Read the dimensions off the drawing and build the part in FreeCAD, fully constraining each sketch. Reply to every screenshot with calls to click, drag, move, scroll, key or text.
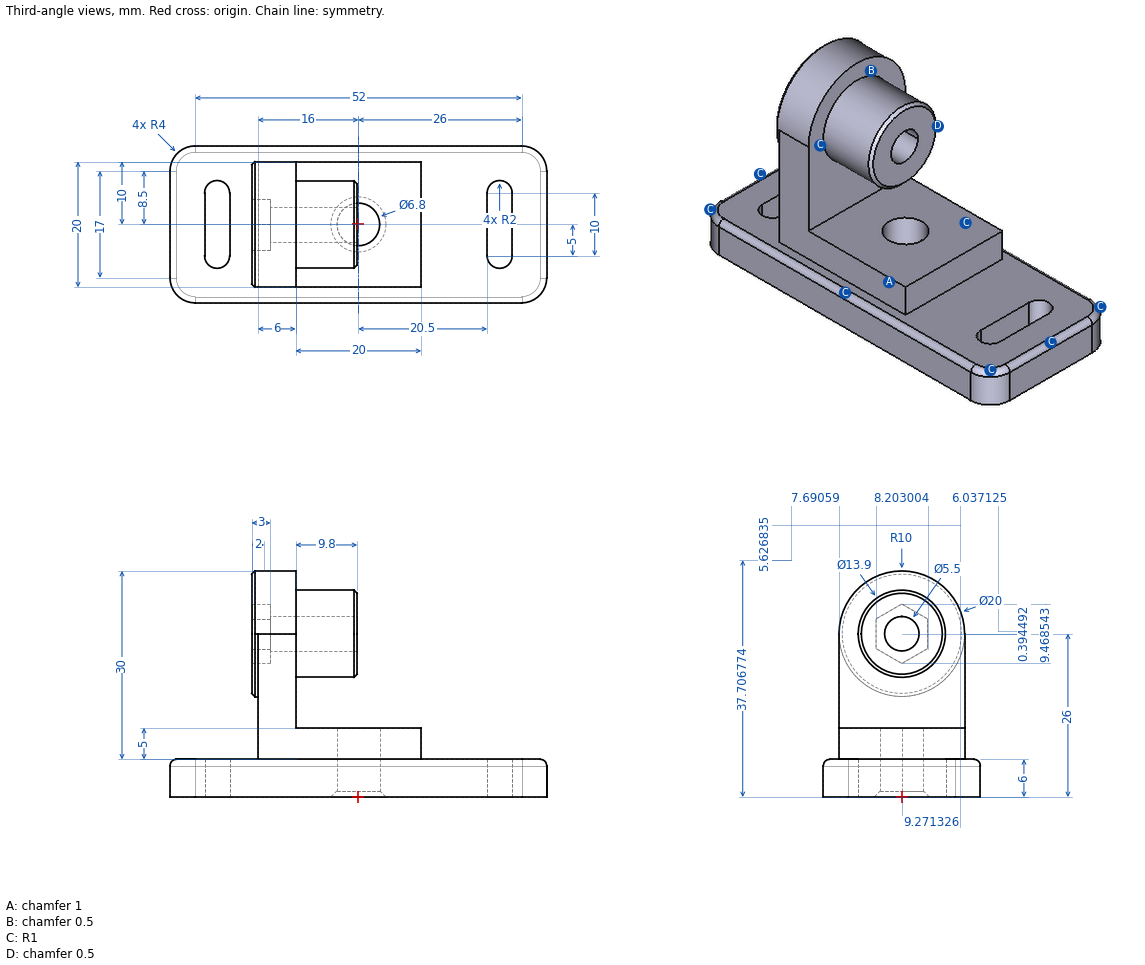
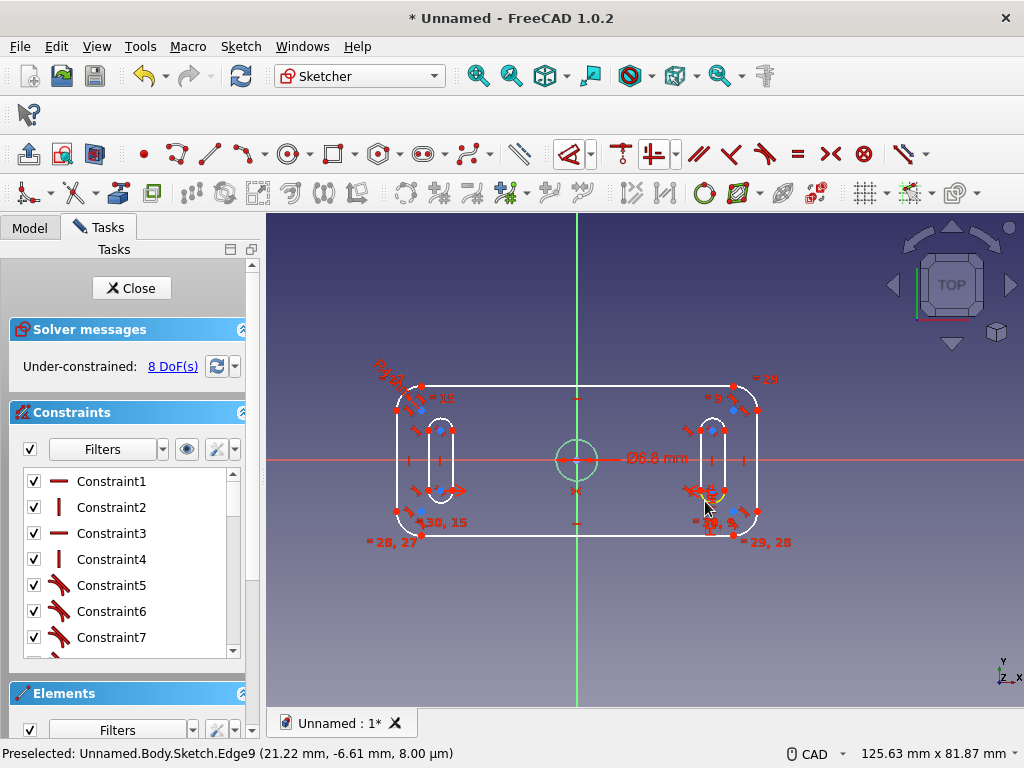
click(639, 386)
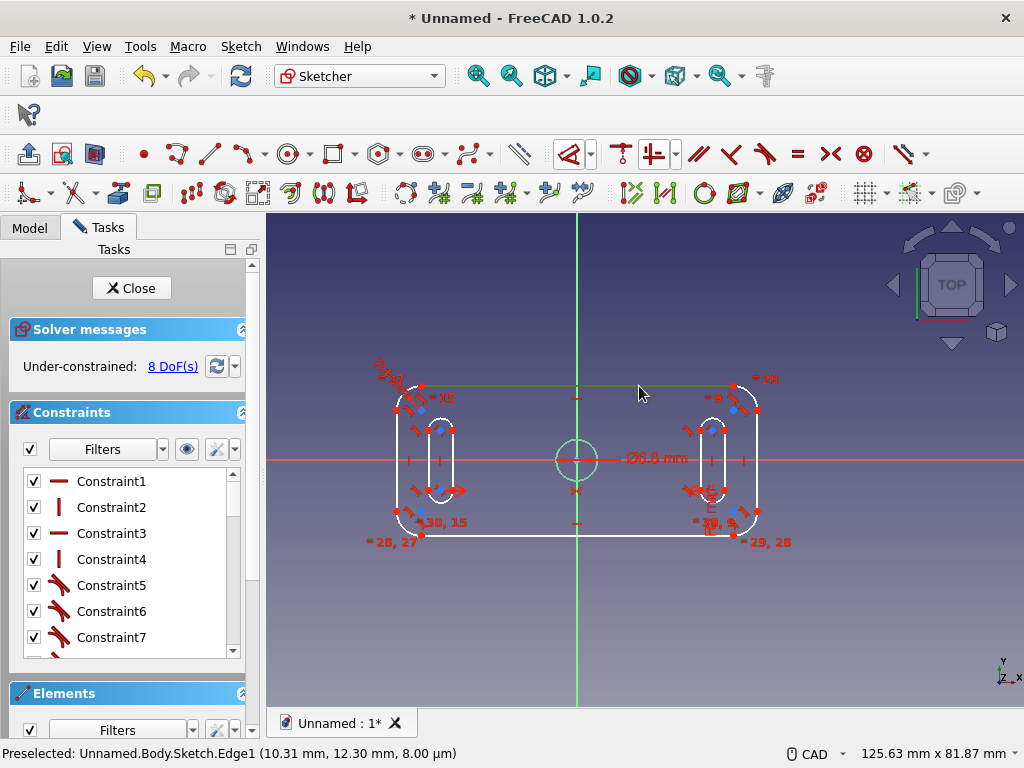
click(590, 154)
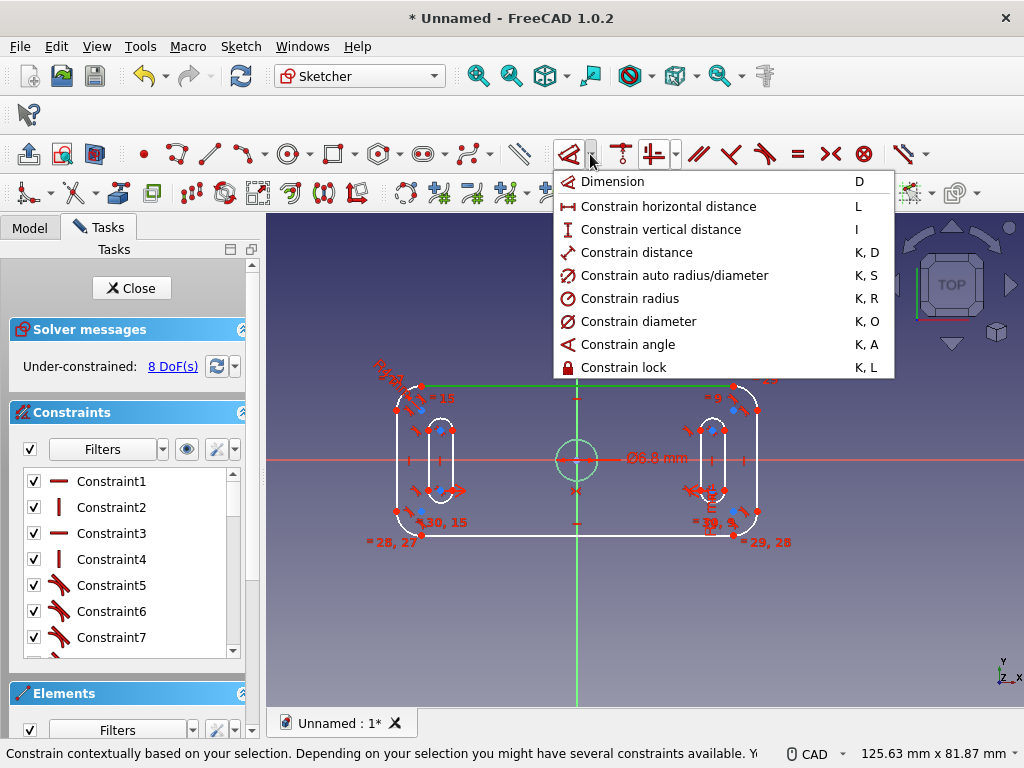
click(724, 206)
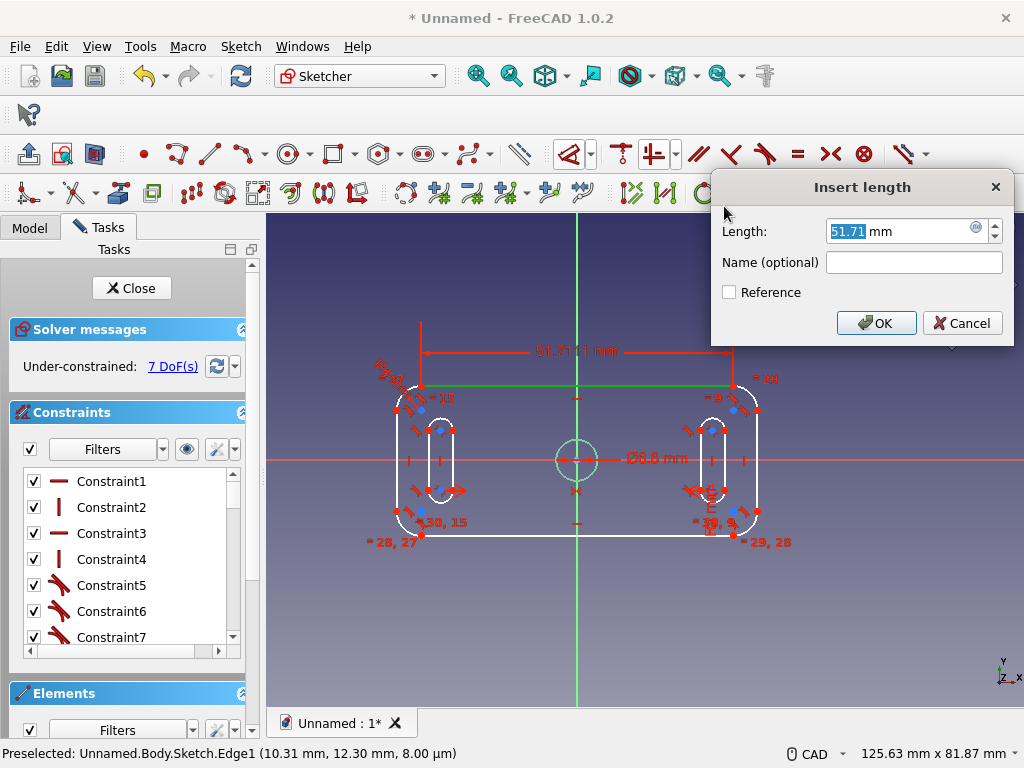
text(52)
key(Return)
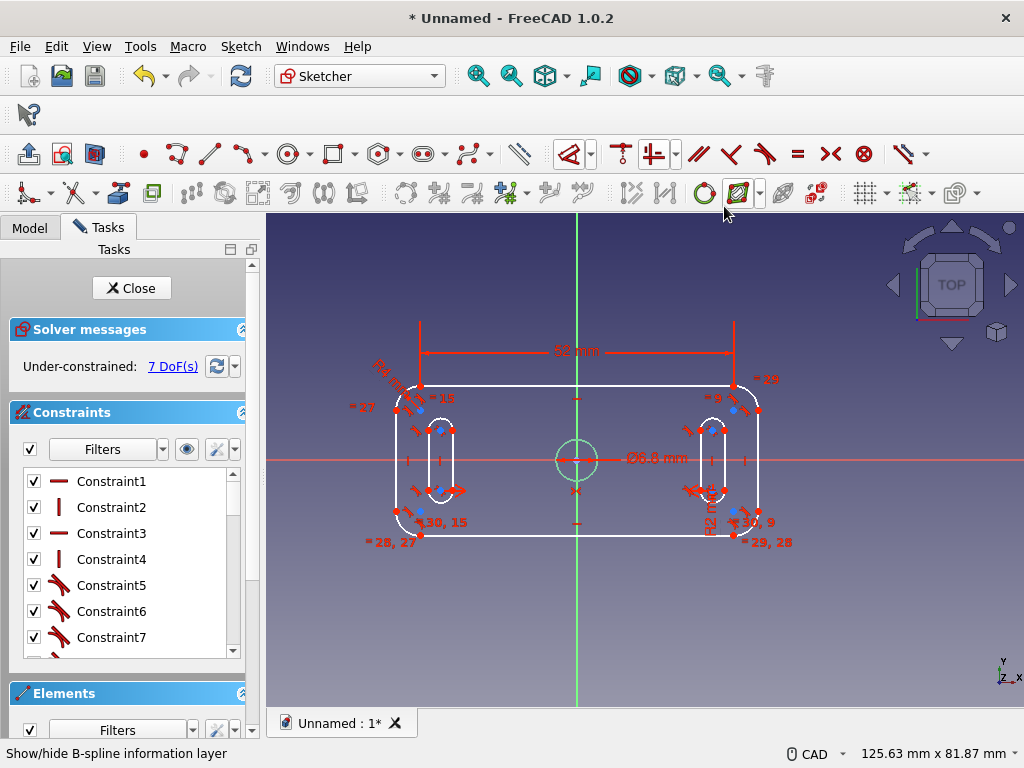
click(396, 441)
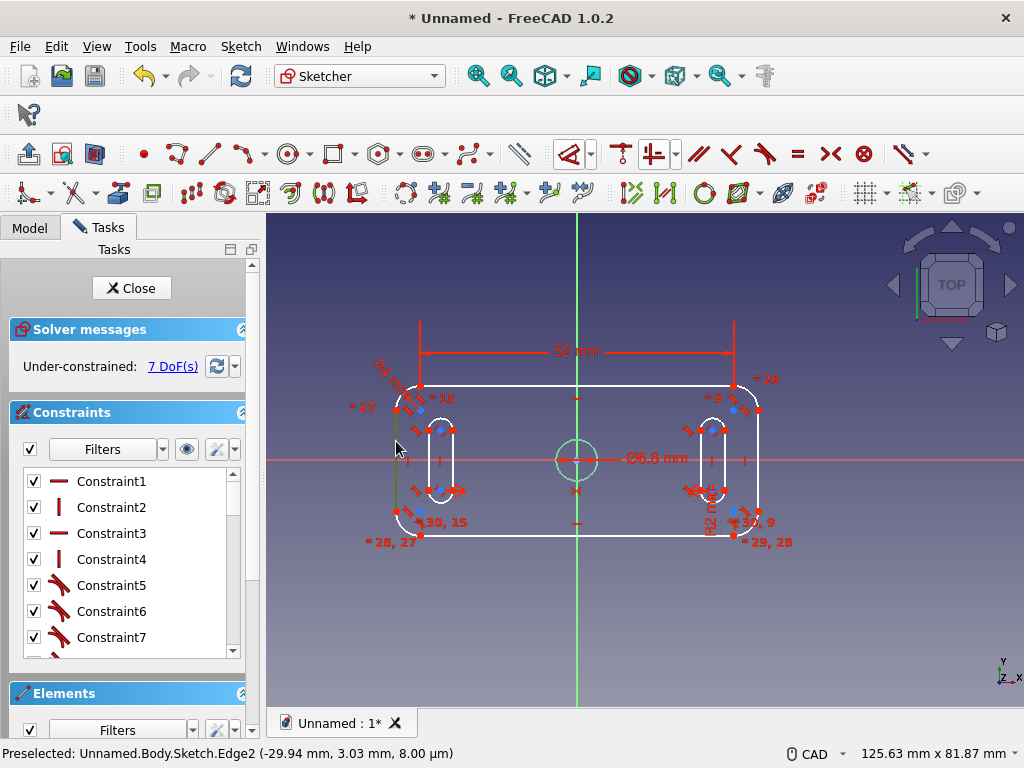
key(i)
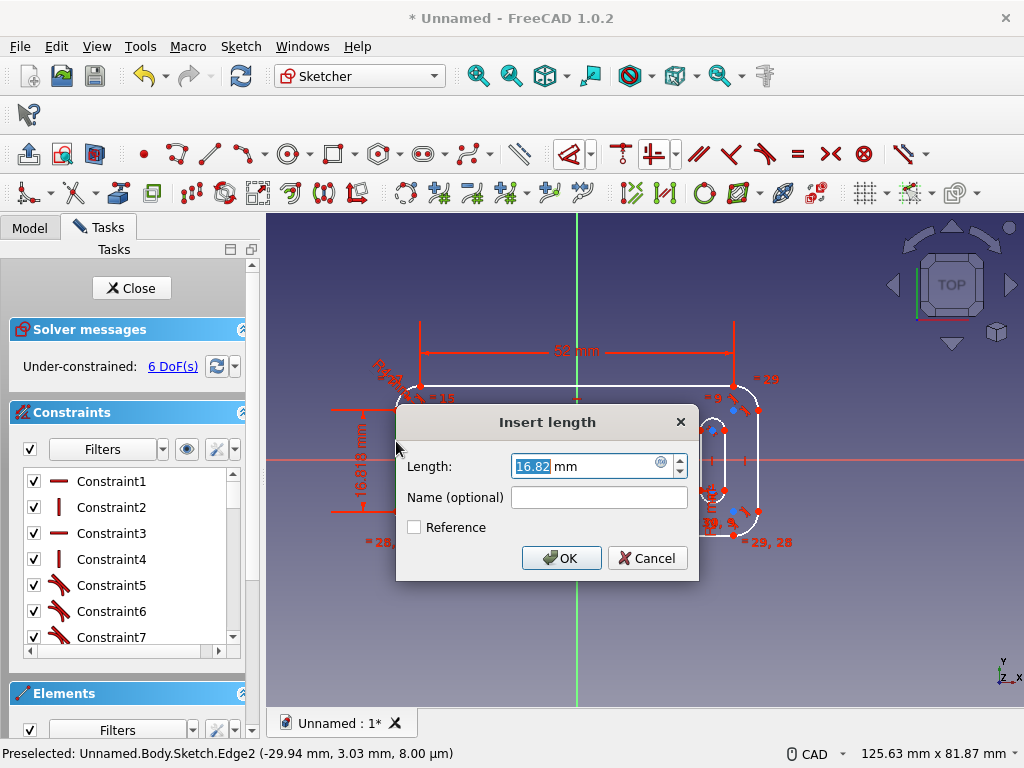
text(17)
key(Return)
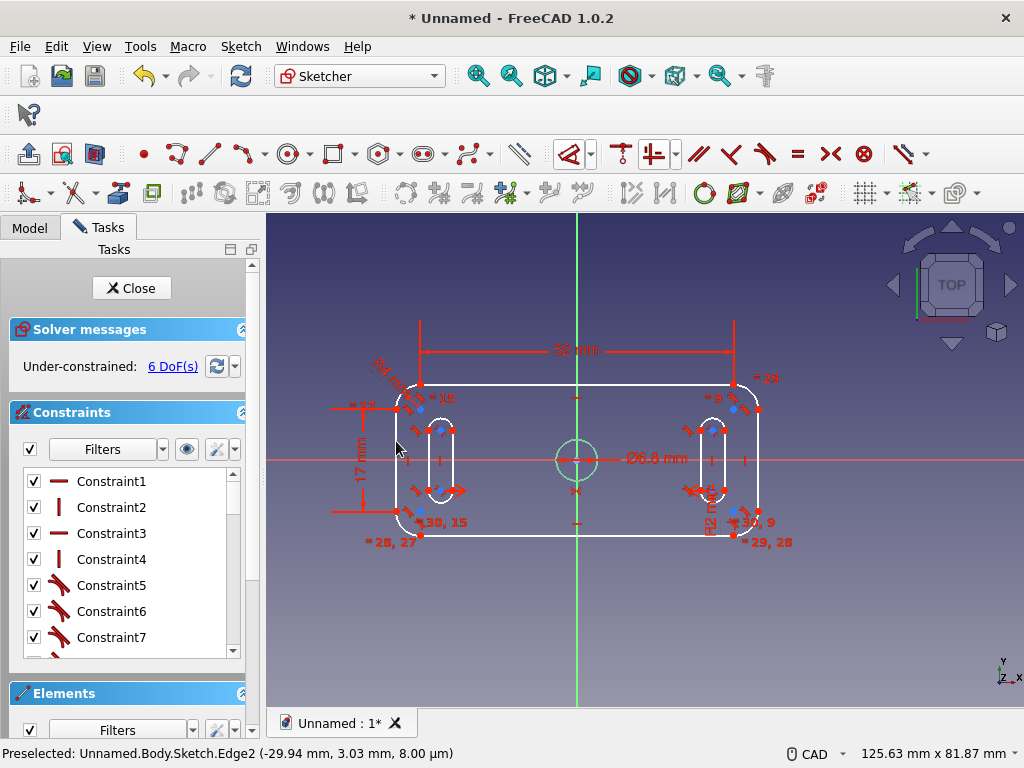
click(701, 473)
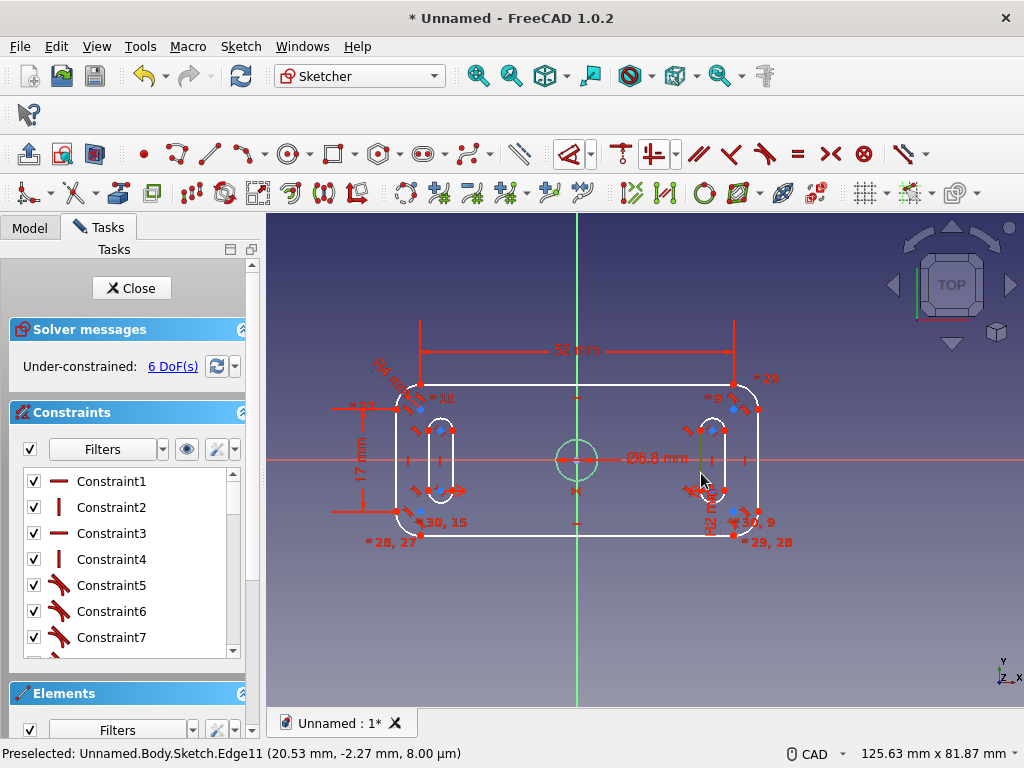
key(i)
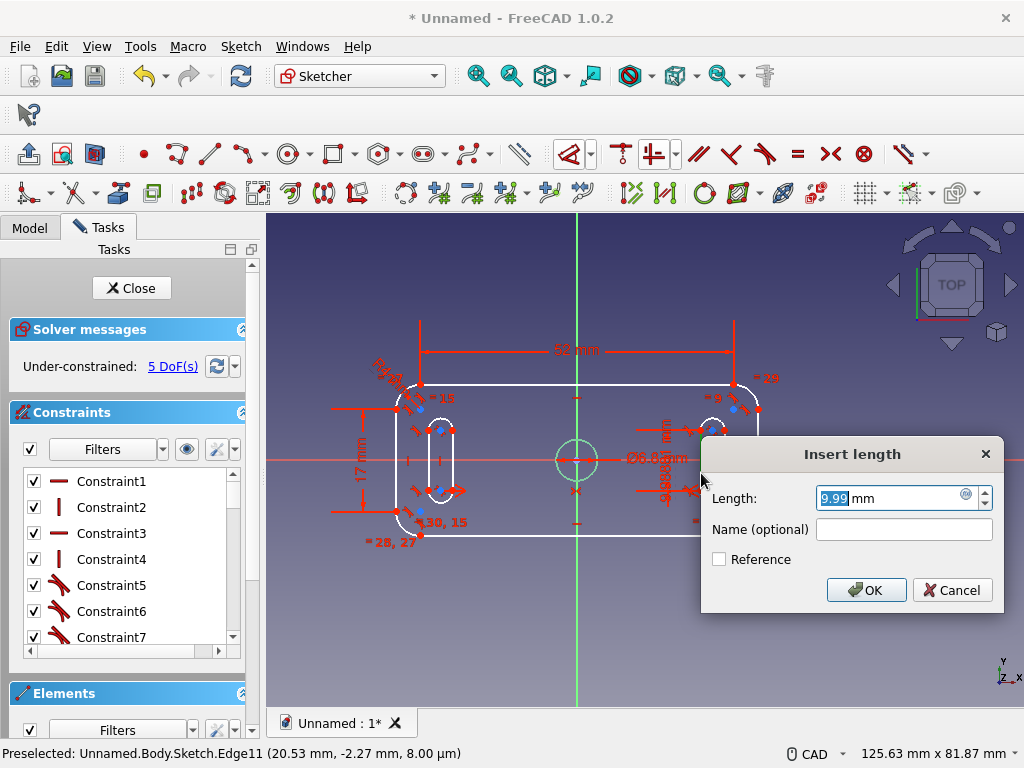
text(10)
key(Return)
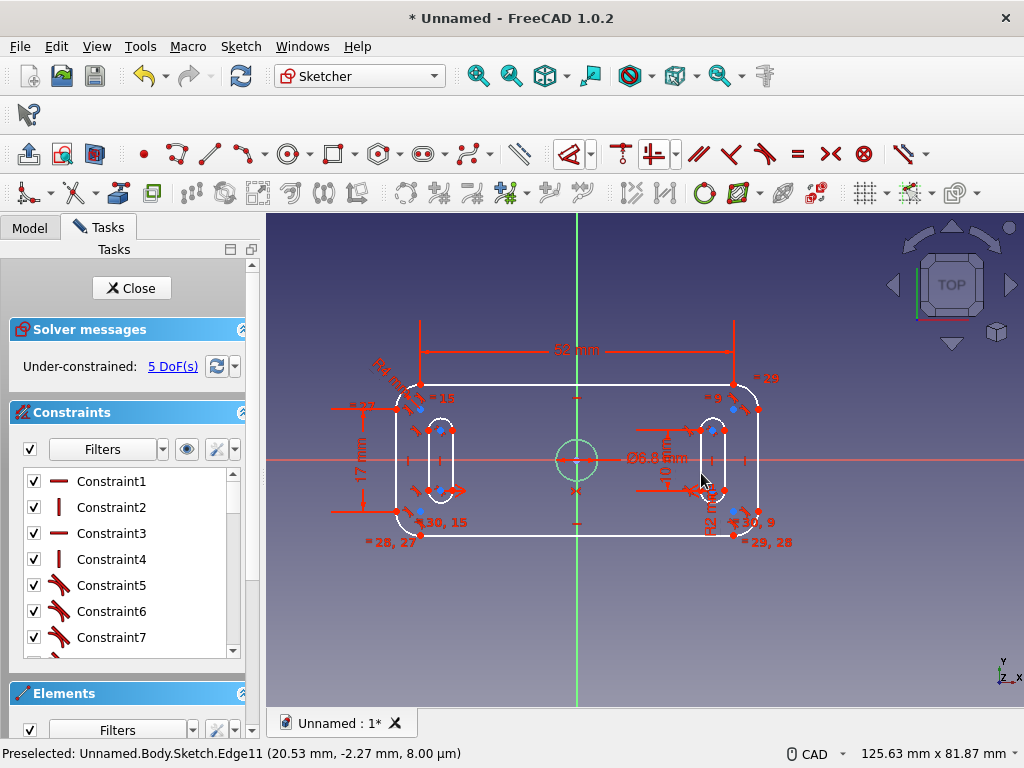
click(429, 473)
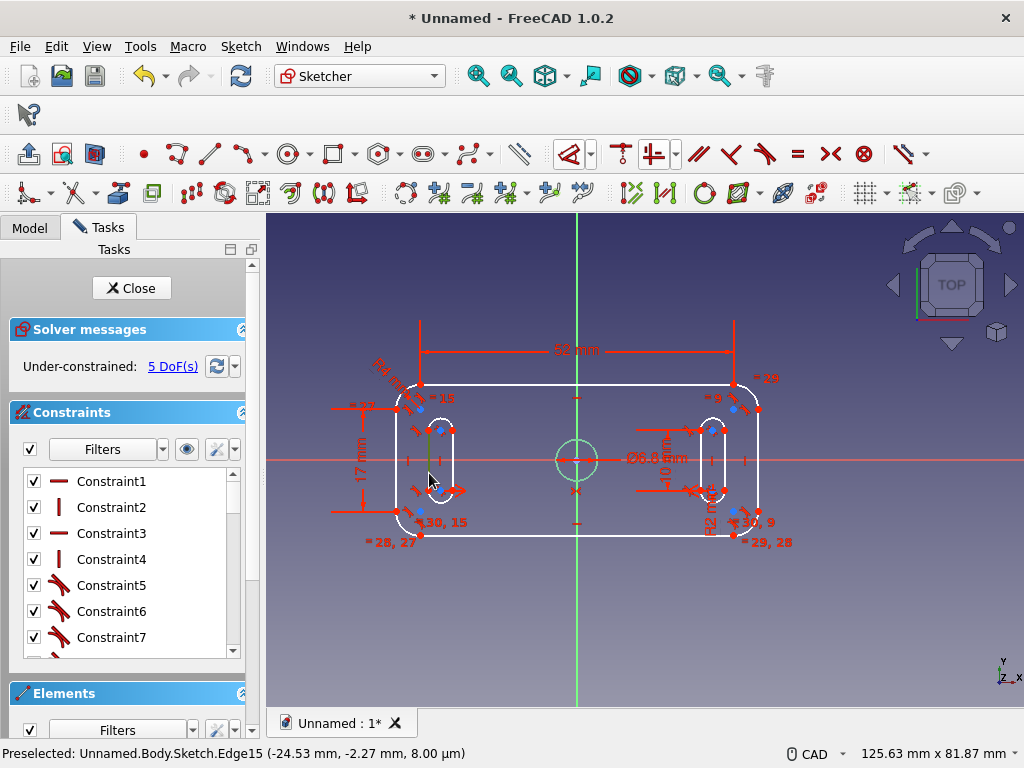
click(590, 154)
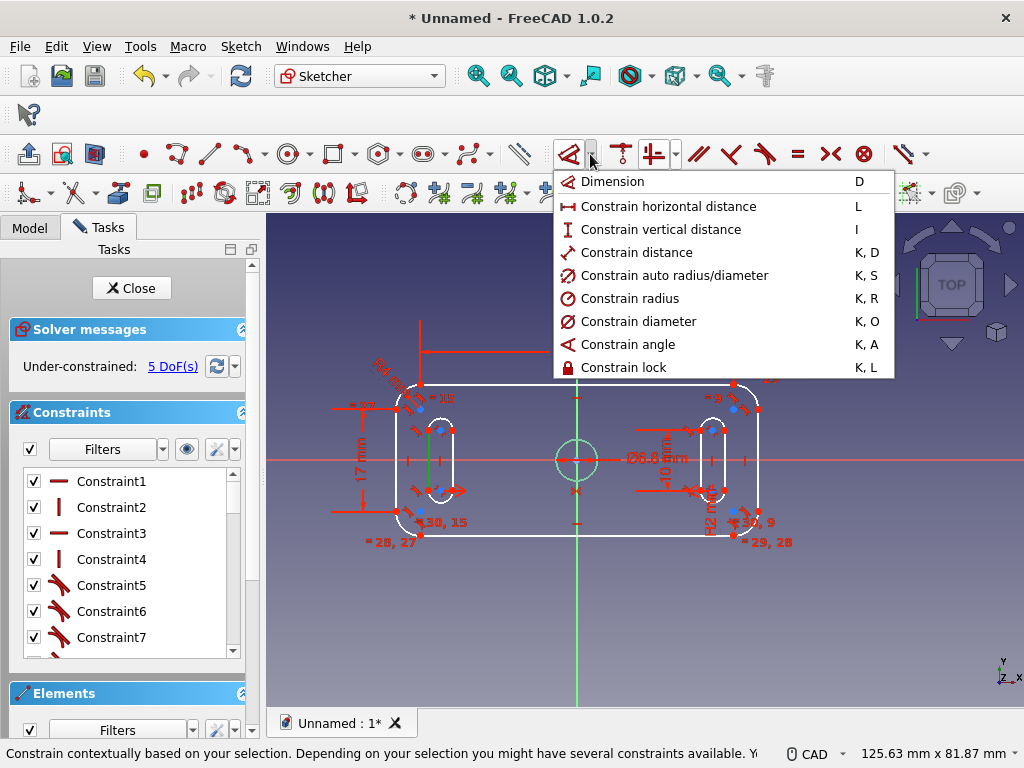
click(724, 230)